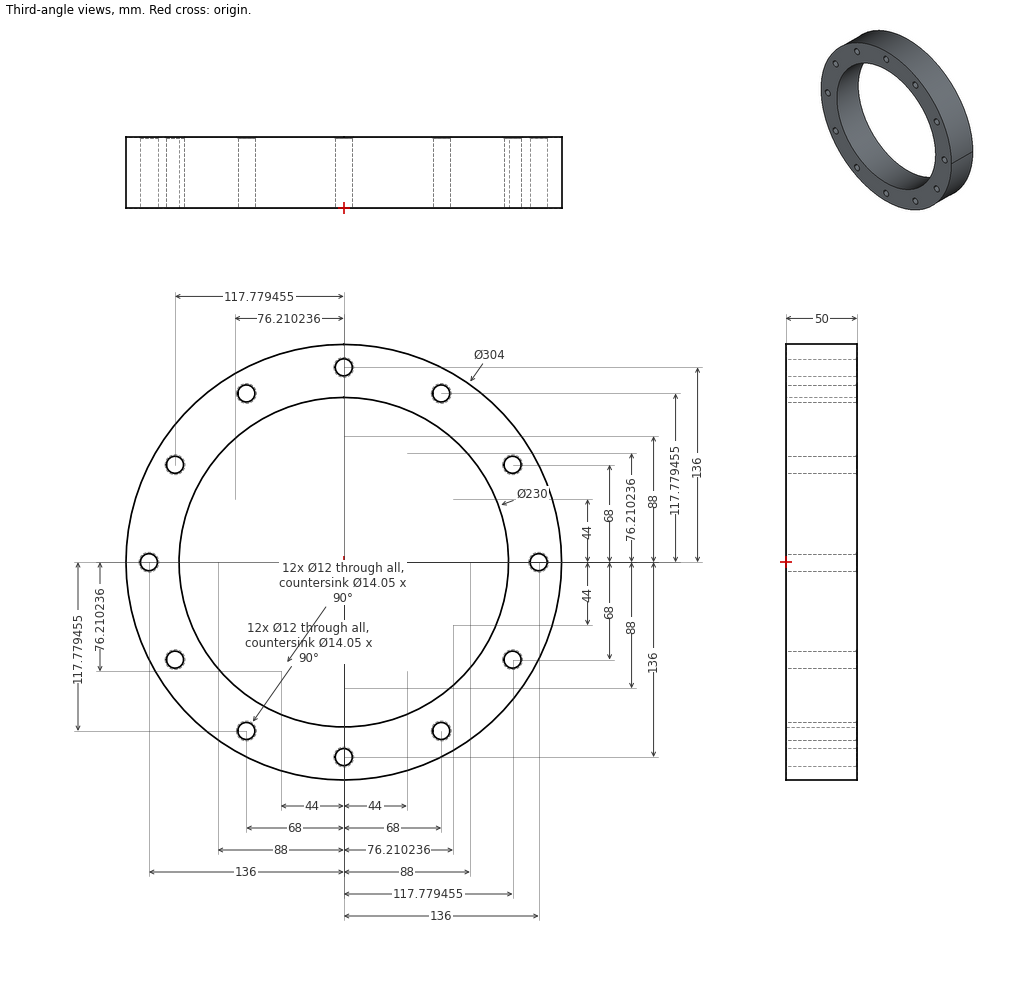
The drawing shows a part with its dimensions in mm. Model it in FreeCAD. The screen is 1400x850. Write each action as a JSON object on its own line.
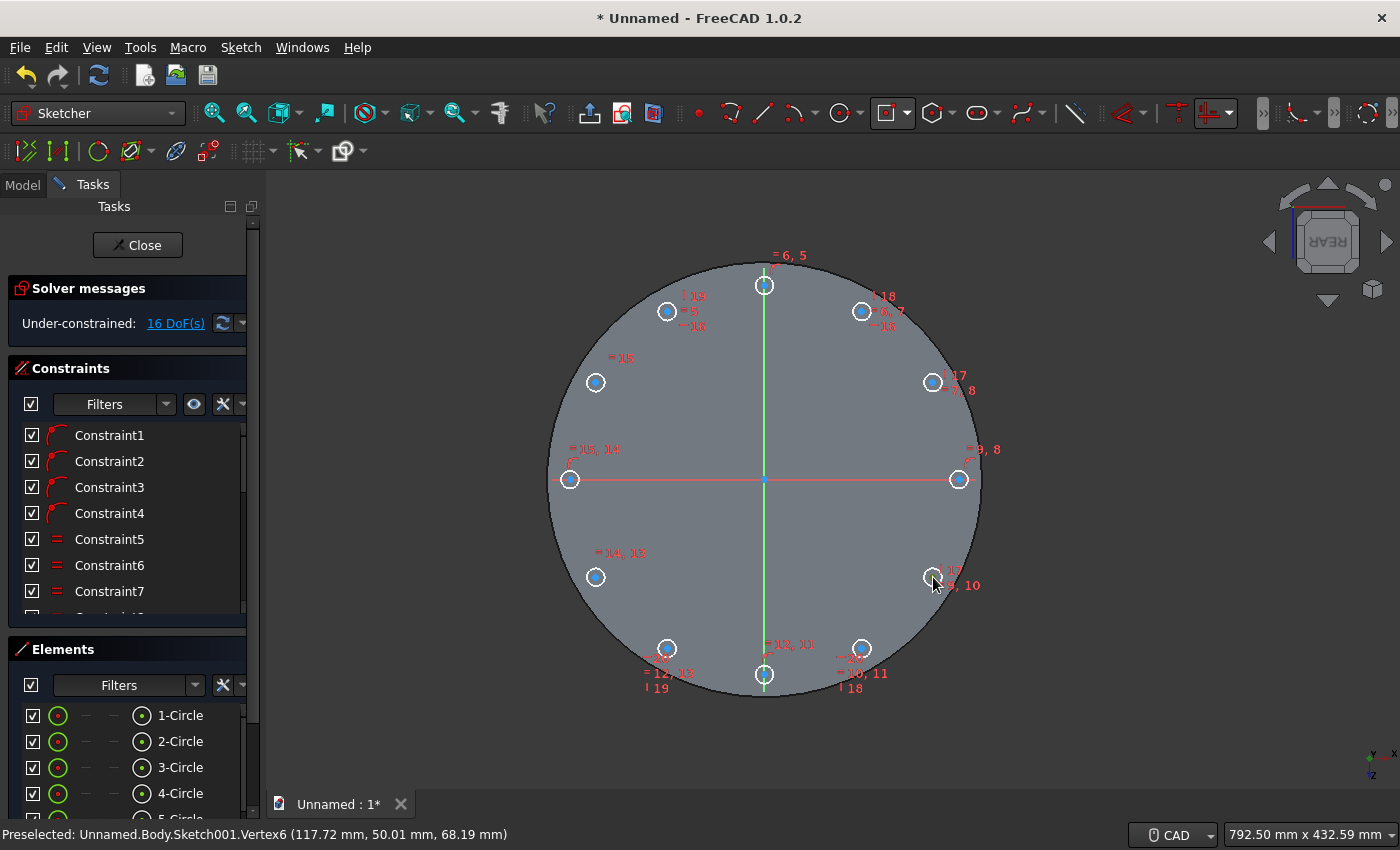
{"action": "left_click", "coordinate": [596, 577]}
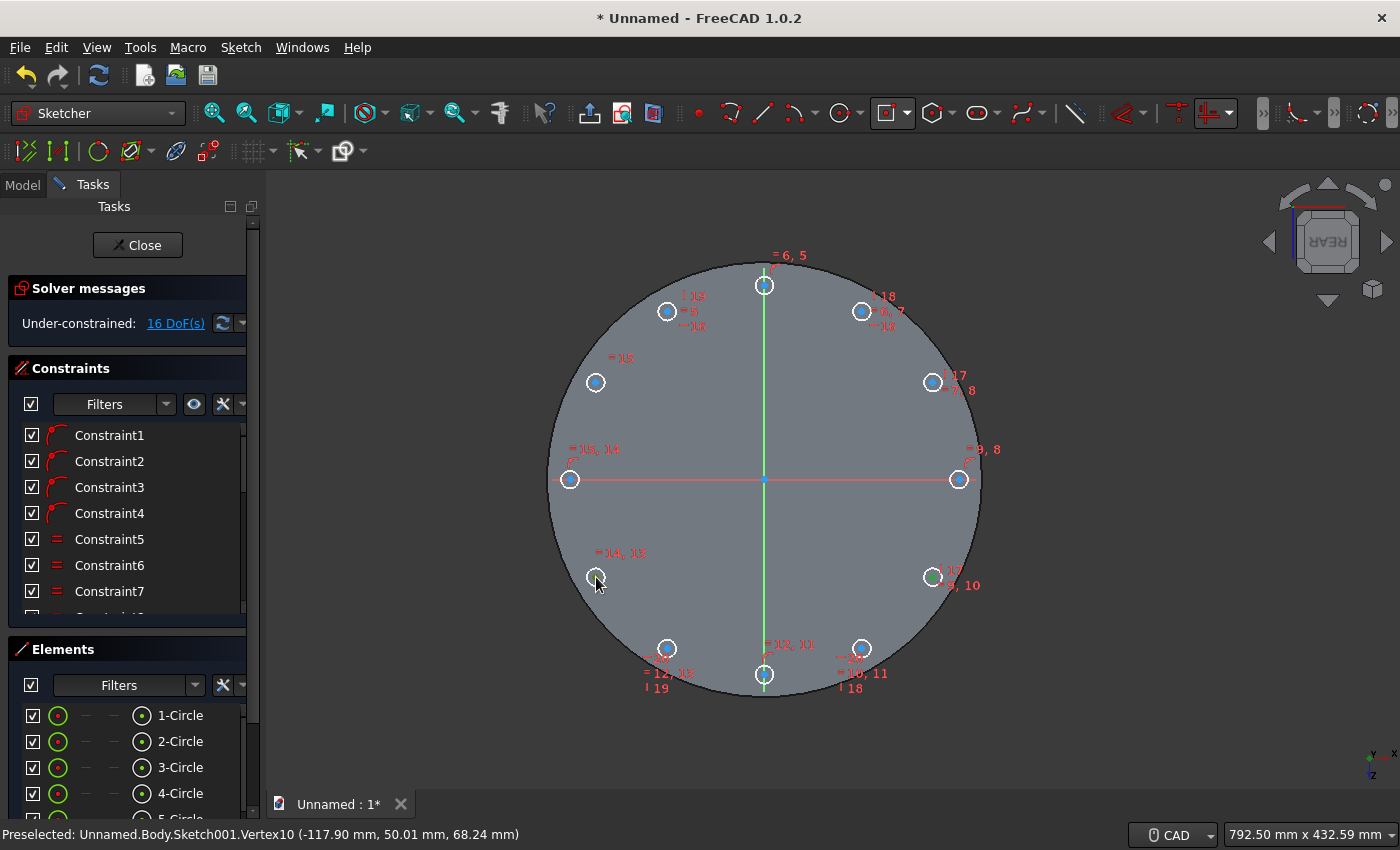
{"action": "left_click", "coordinate": [1232, 114]}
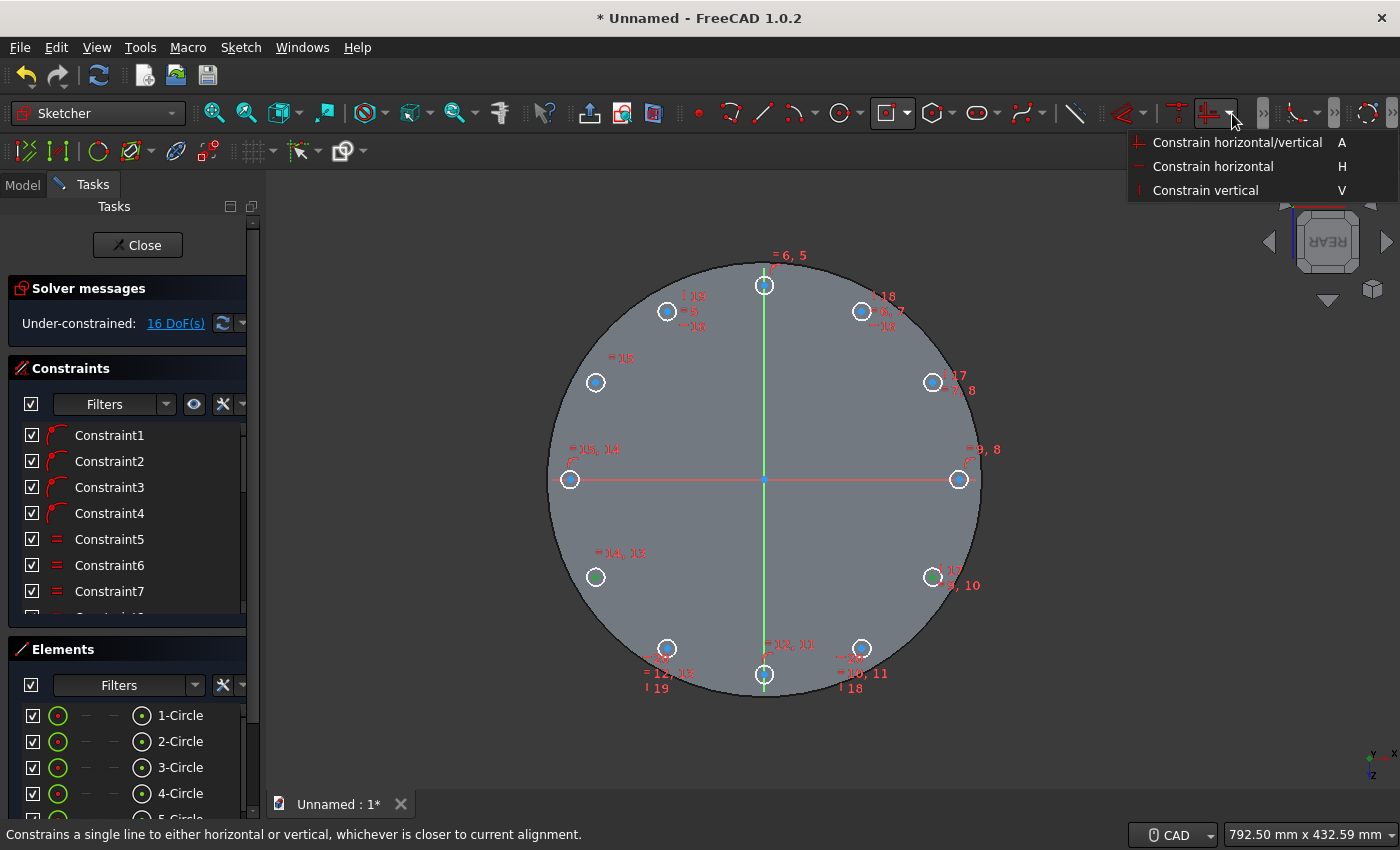
{"action": "left_click", "coordinate": [1263, 166]}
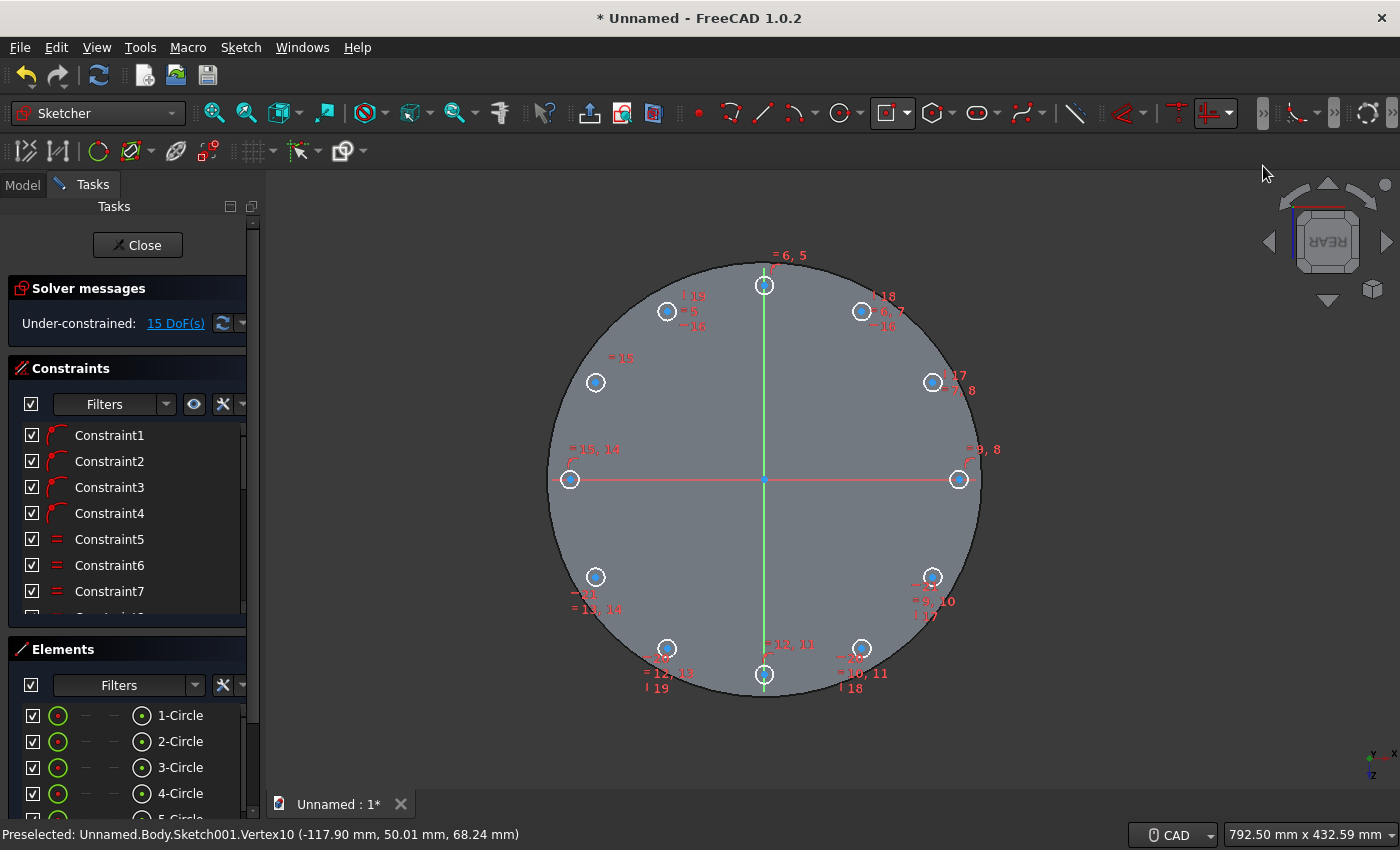
{"action": "left_click", "coordinate": [596, 577]}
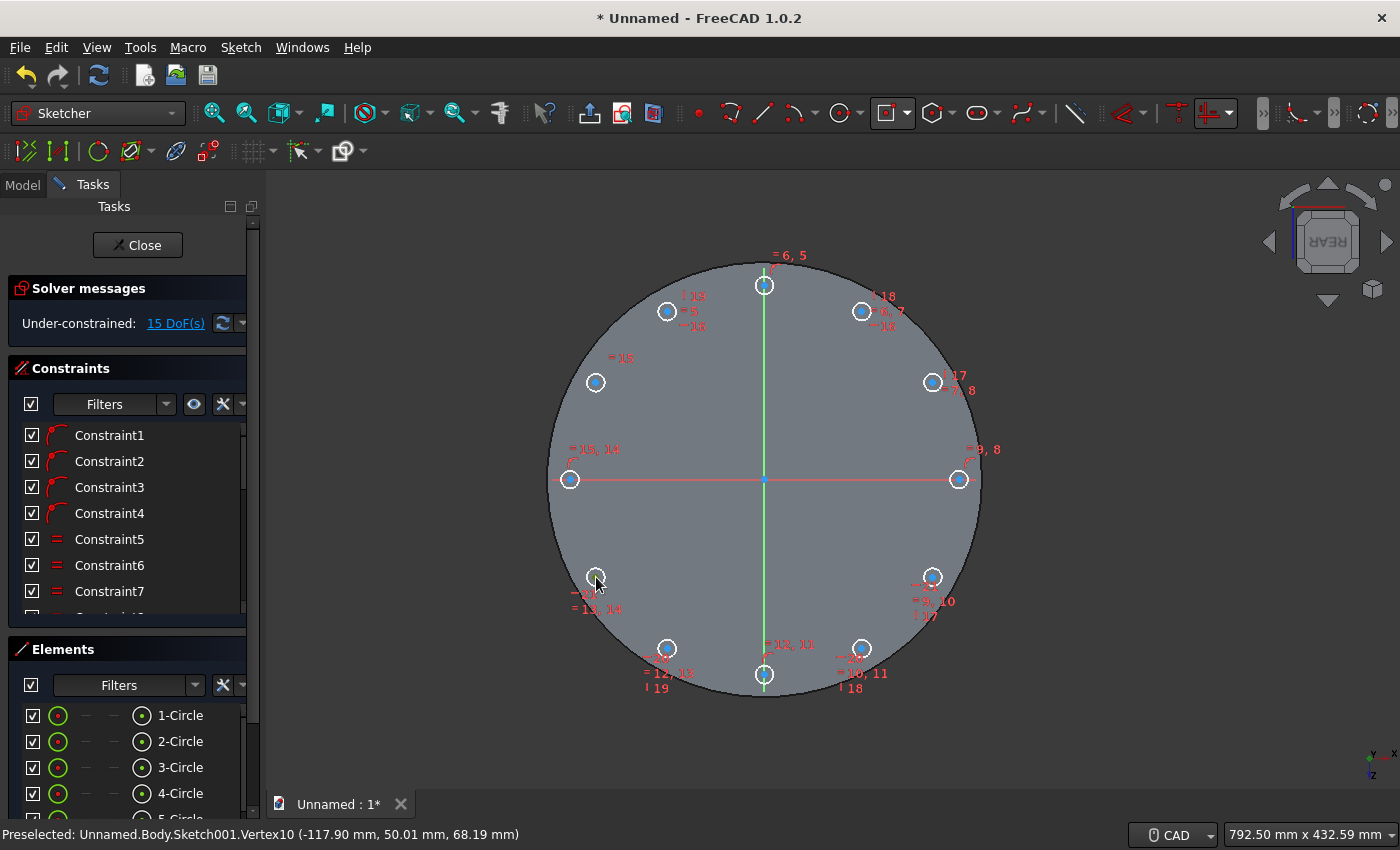
{"action": "left_click", "coordinate": [596, 383]}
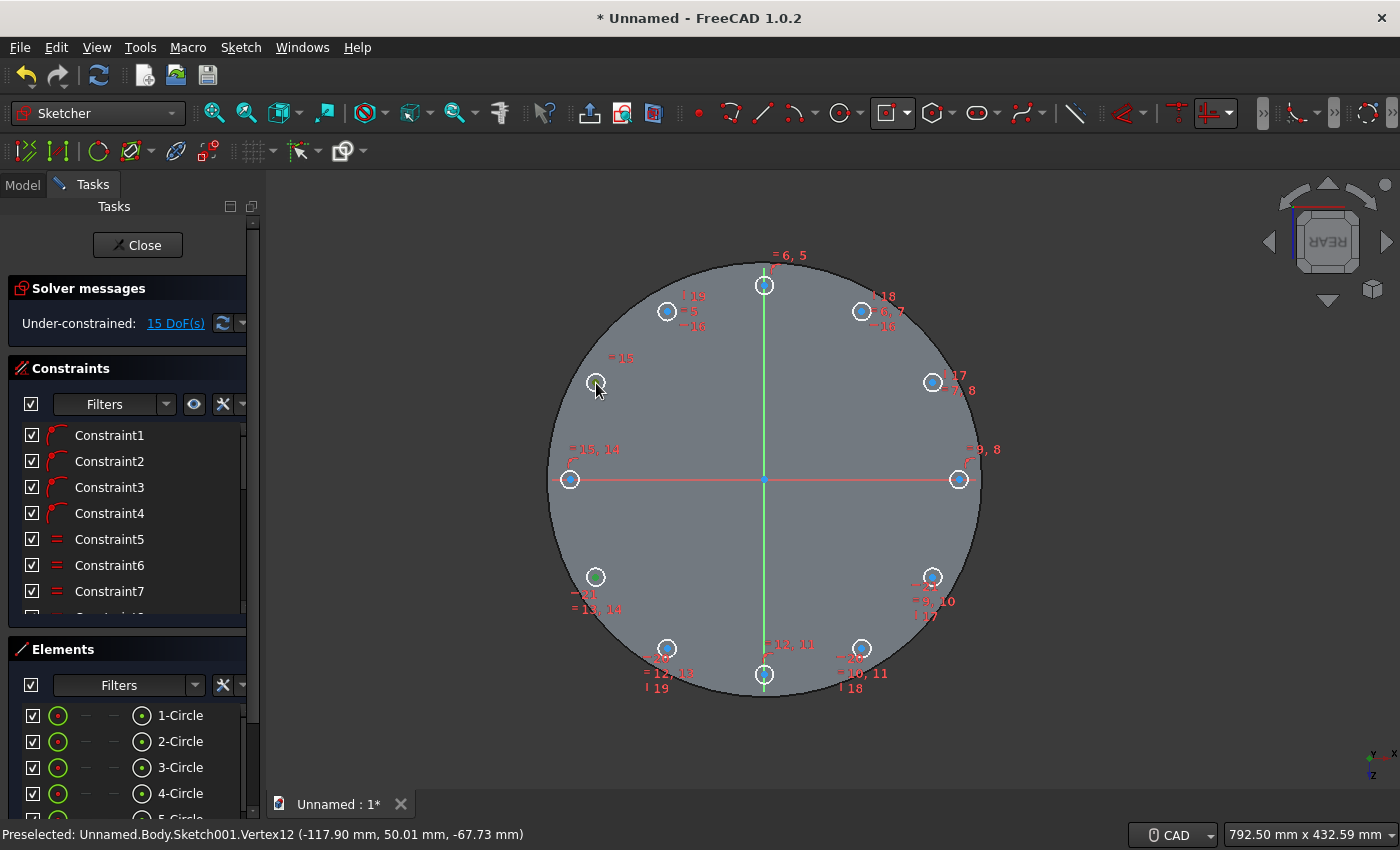
{"action": "key", "text": "v"}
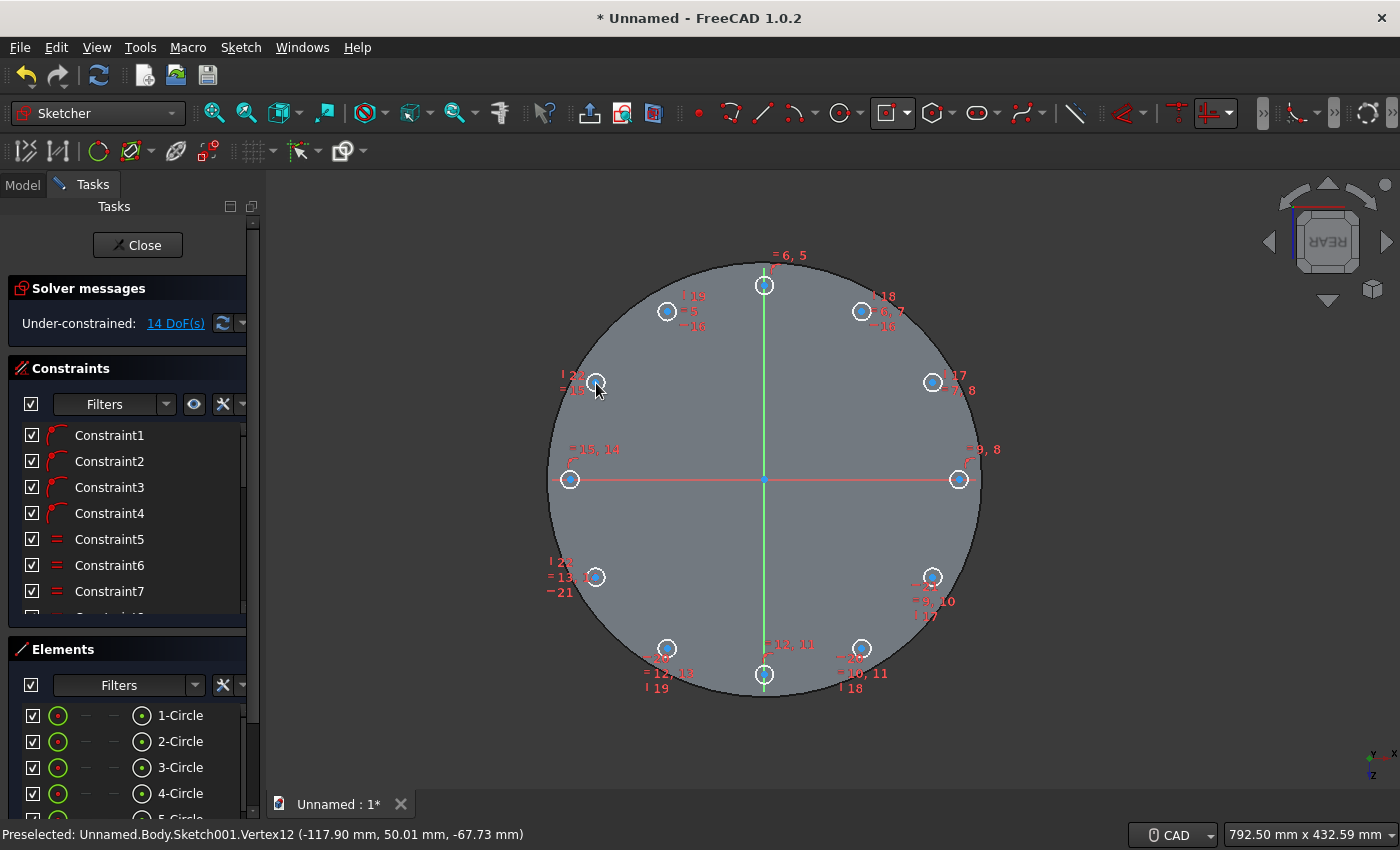
{"action": "left_click", "coordinate": [1122, 114]}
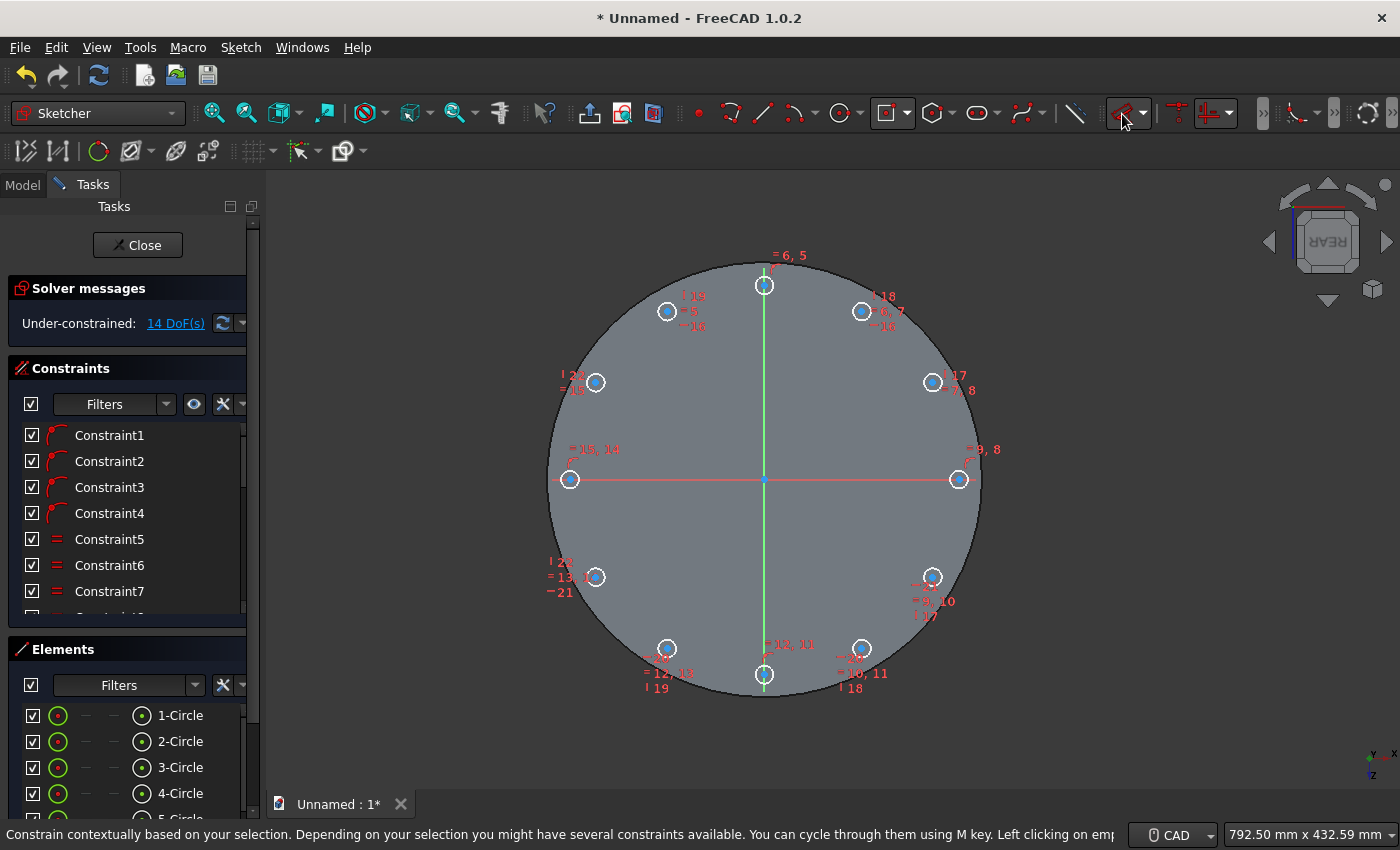
{"action": "scroll", "coordinate": [667, 303], "scroll_direction": "up", "scroll_amount": 5}